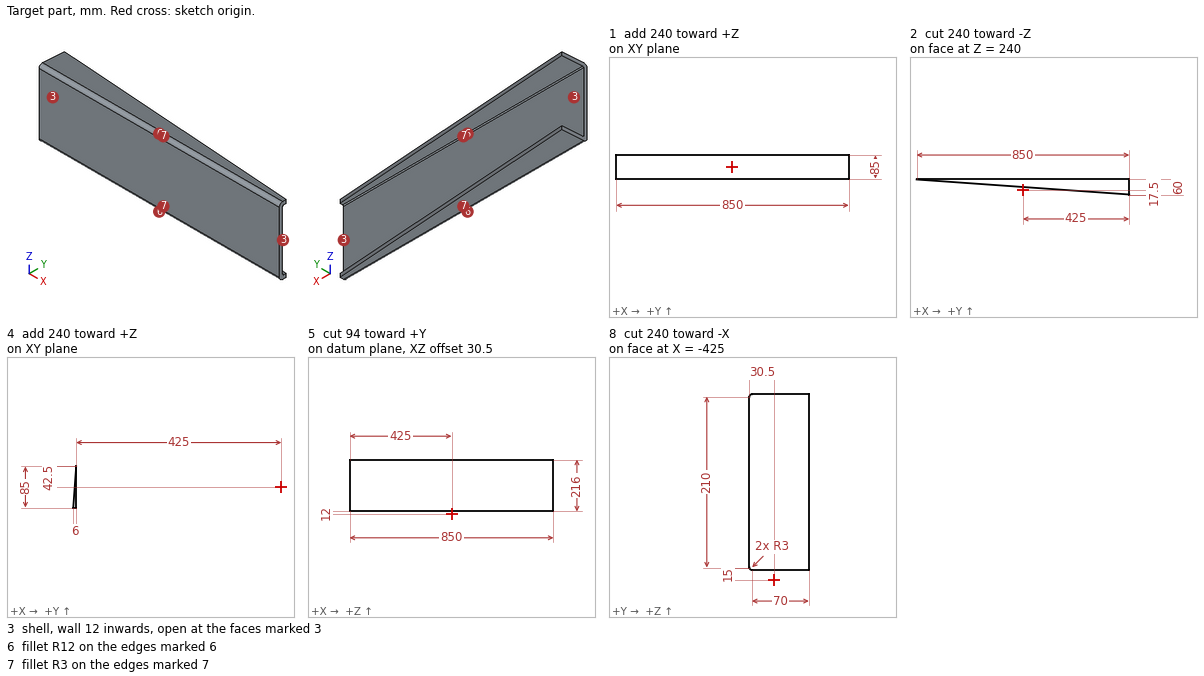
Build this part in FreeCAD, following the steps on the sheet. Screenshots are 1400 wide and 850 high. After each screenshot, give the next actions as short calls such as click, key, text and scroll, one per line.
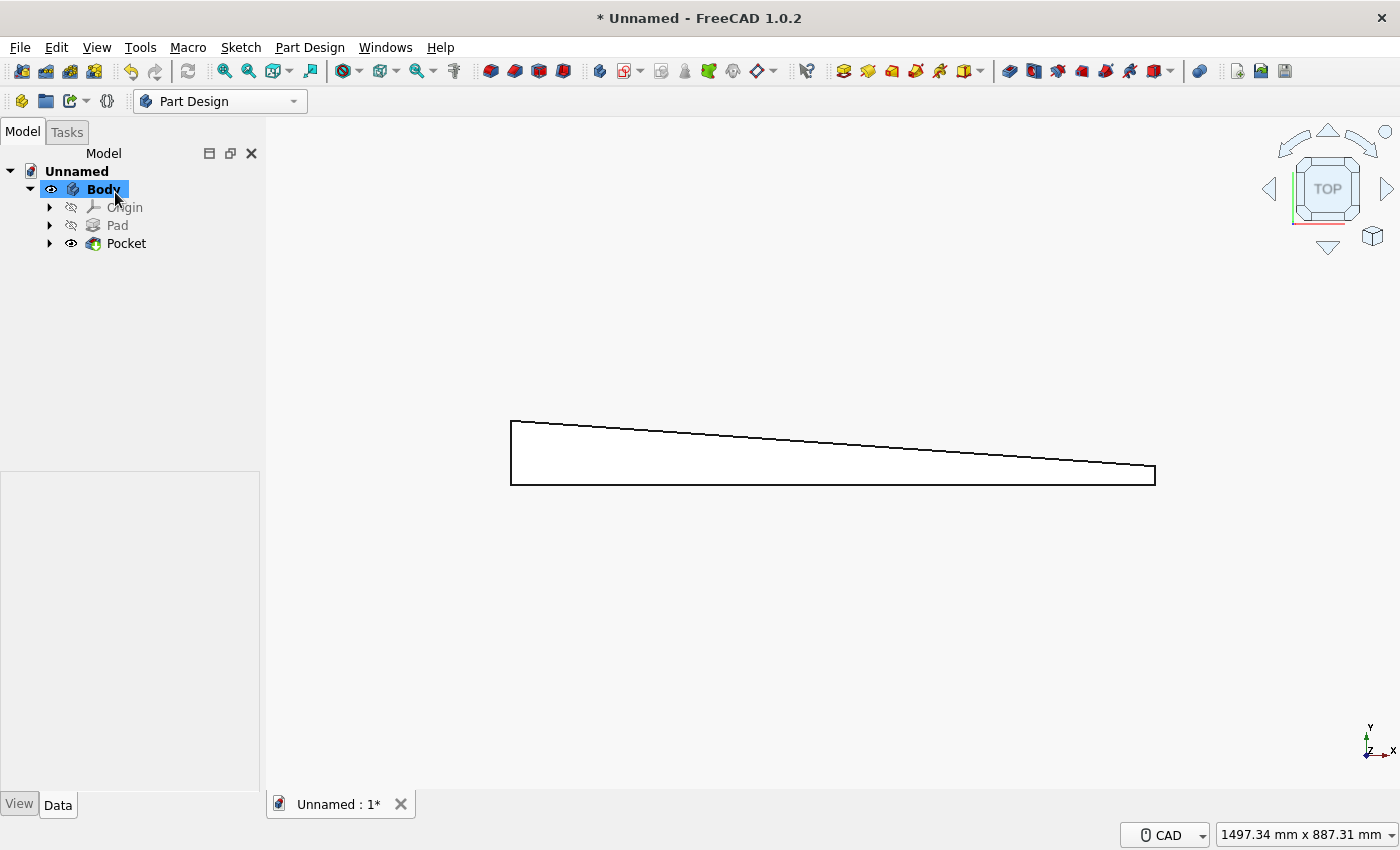
key(1)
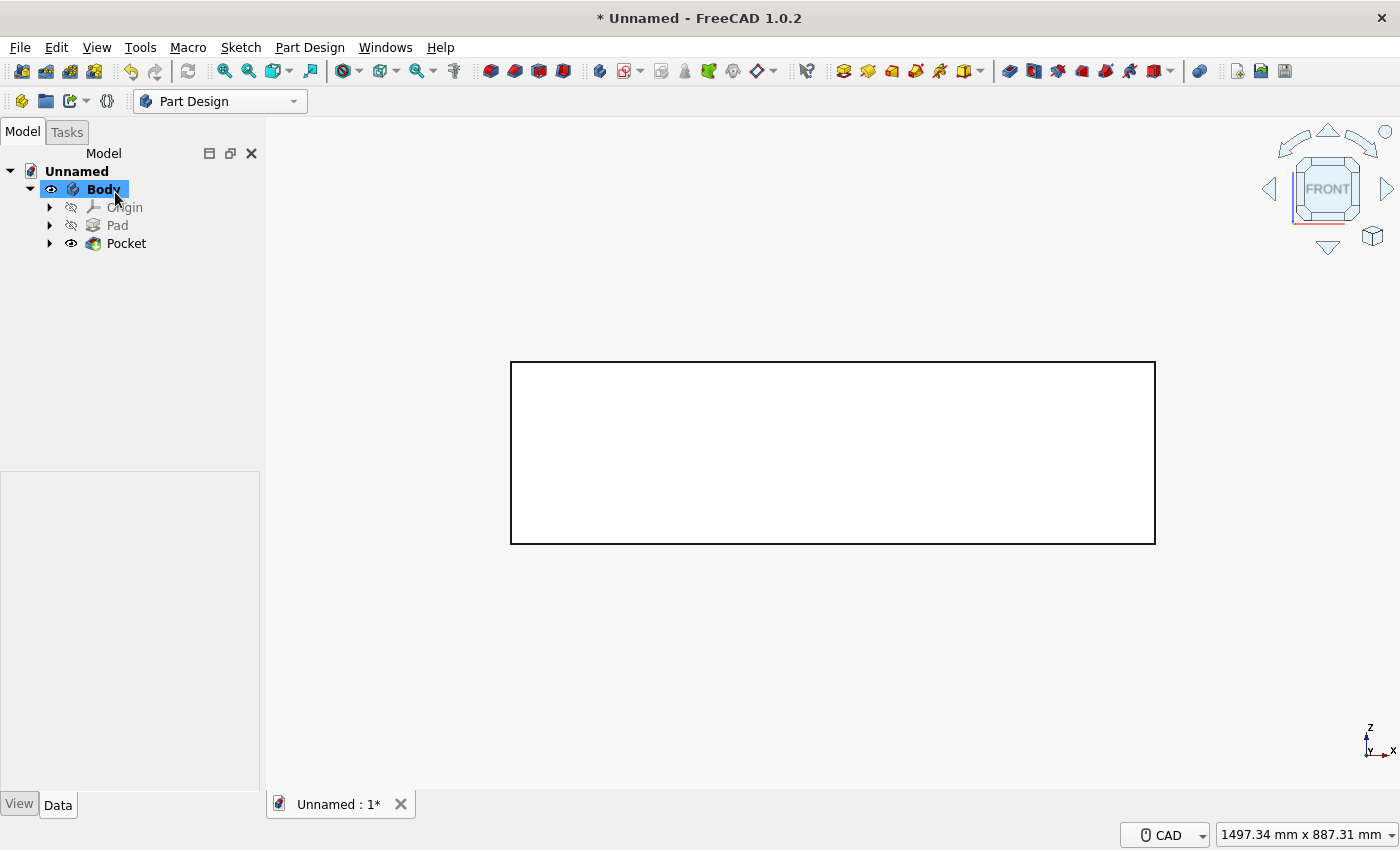
key(3)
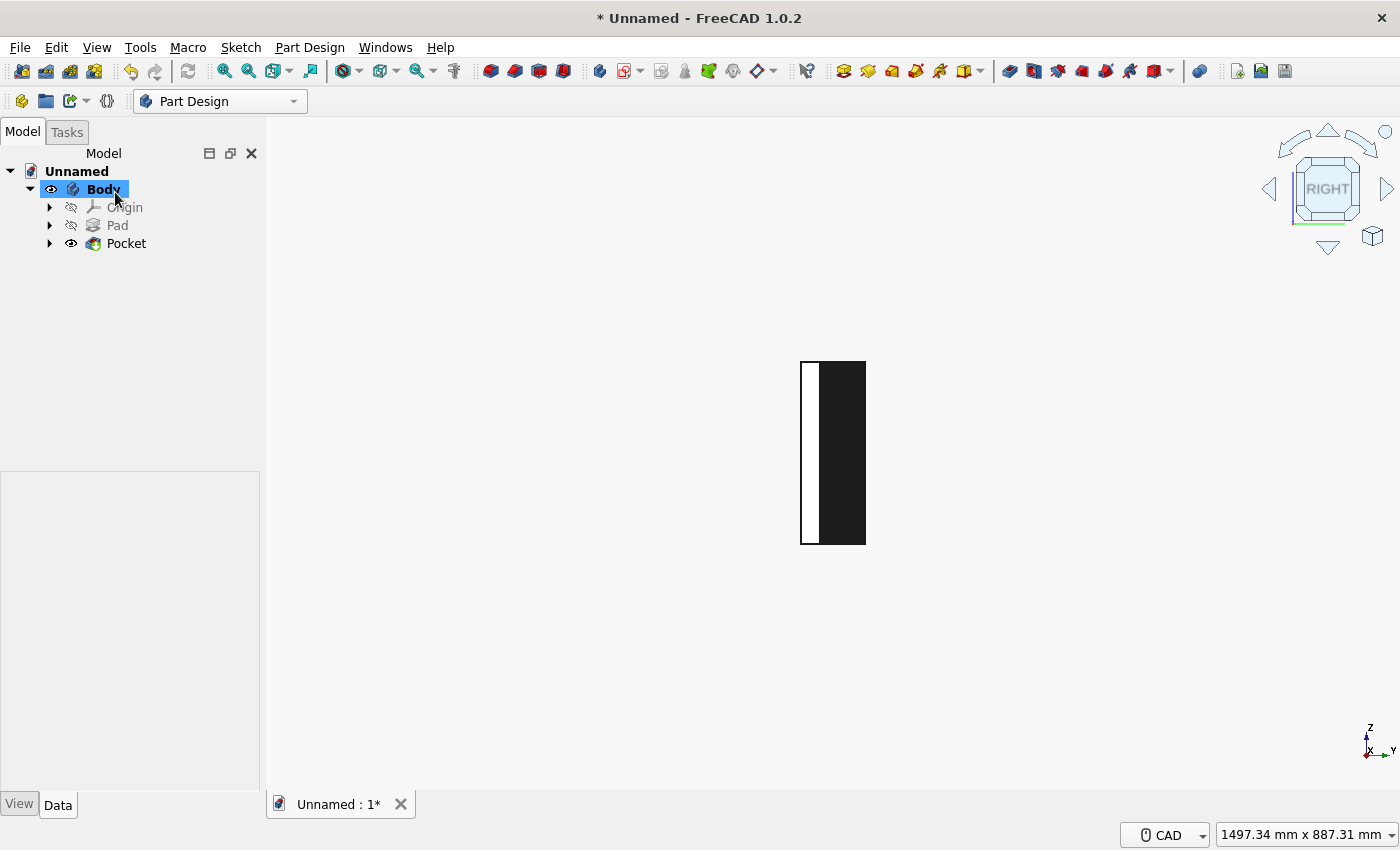
key(v)
key(f)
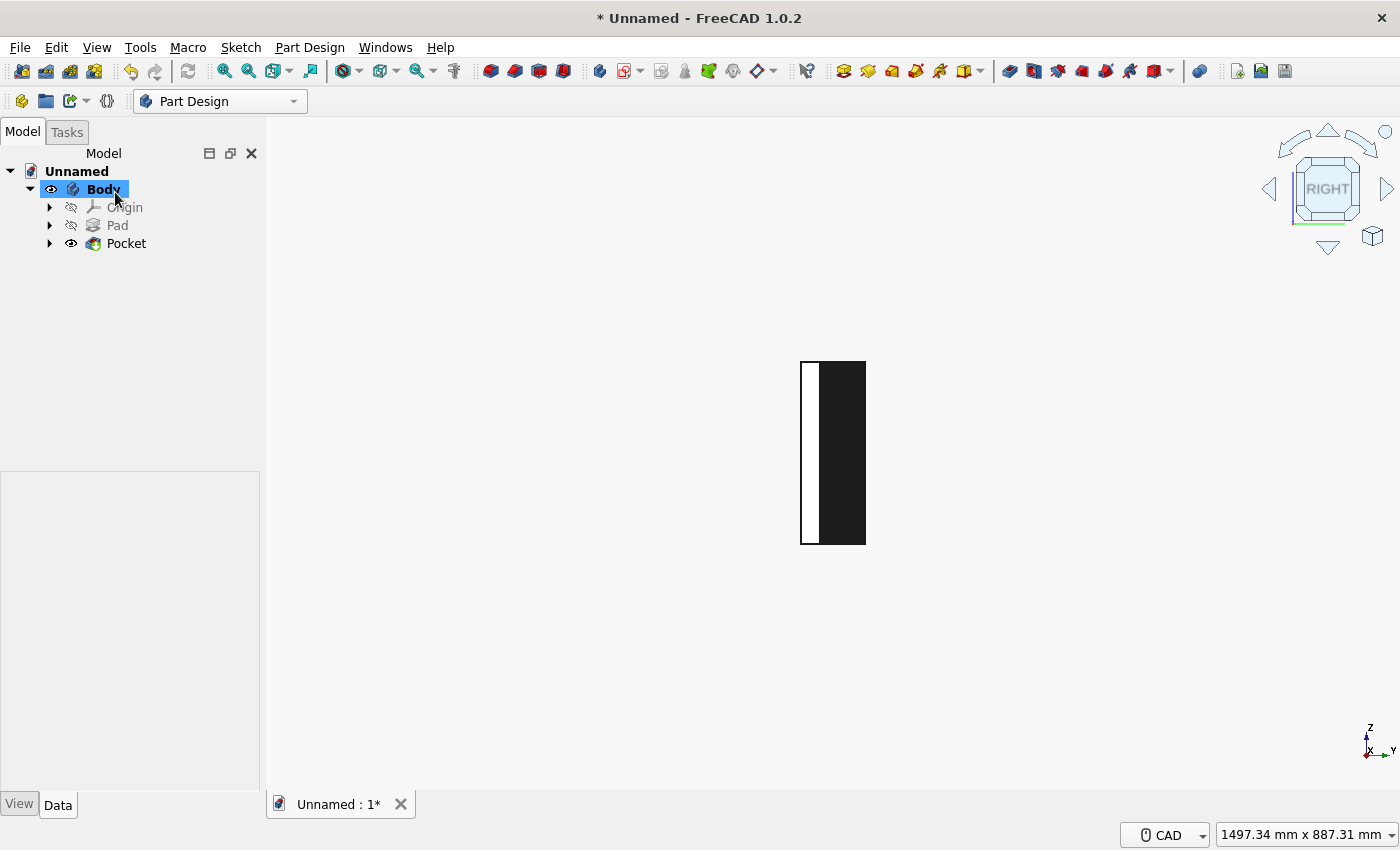
click(810, 374)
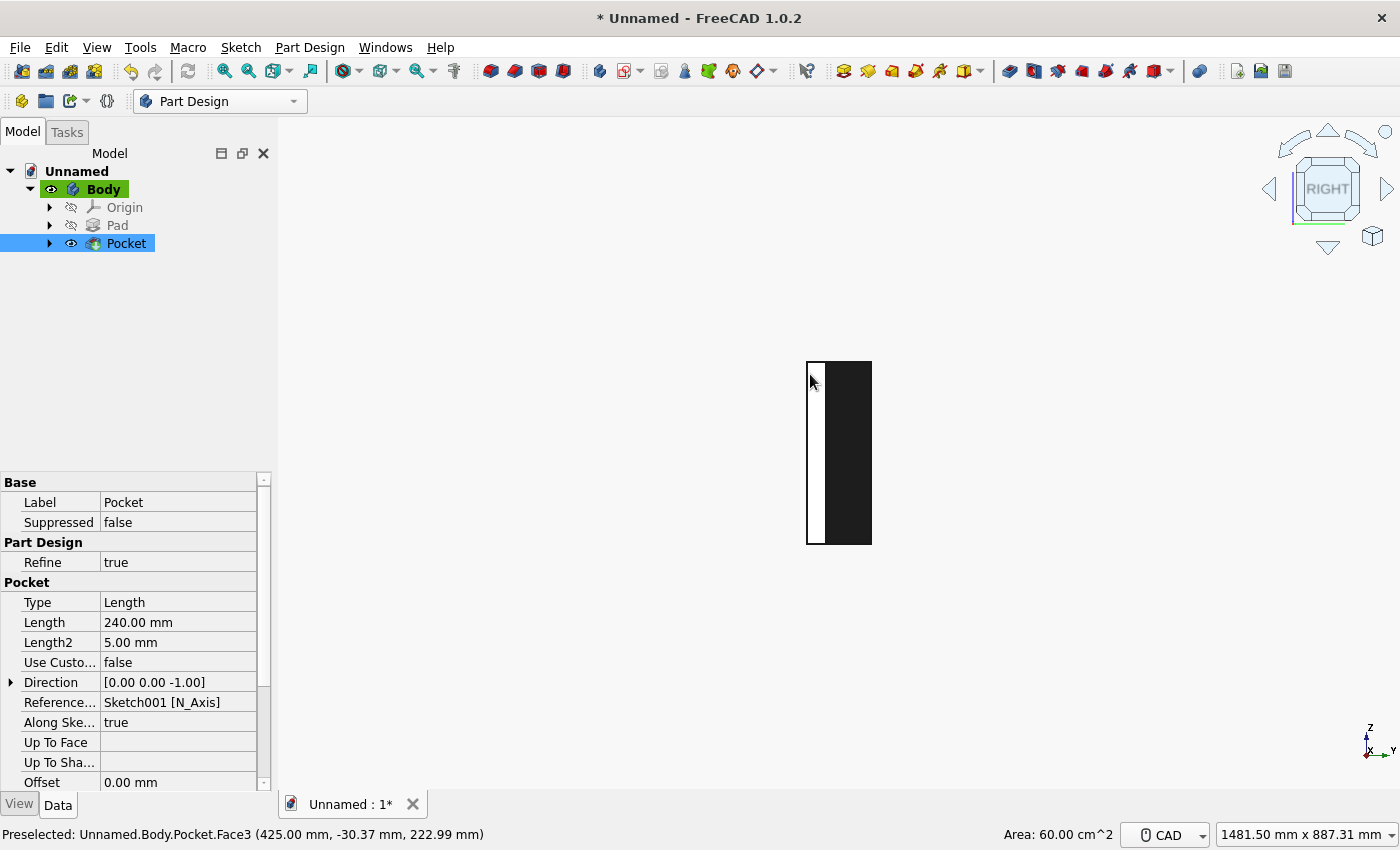
key(5)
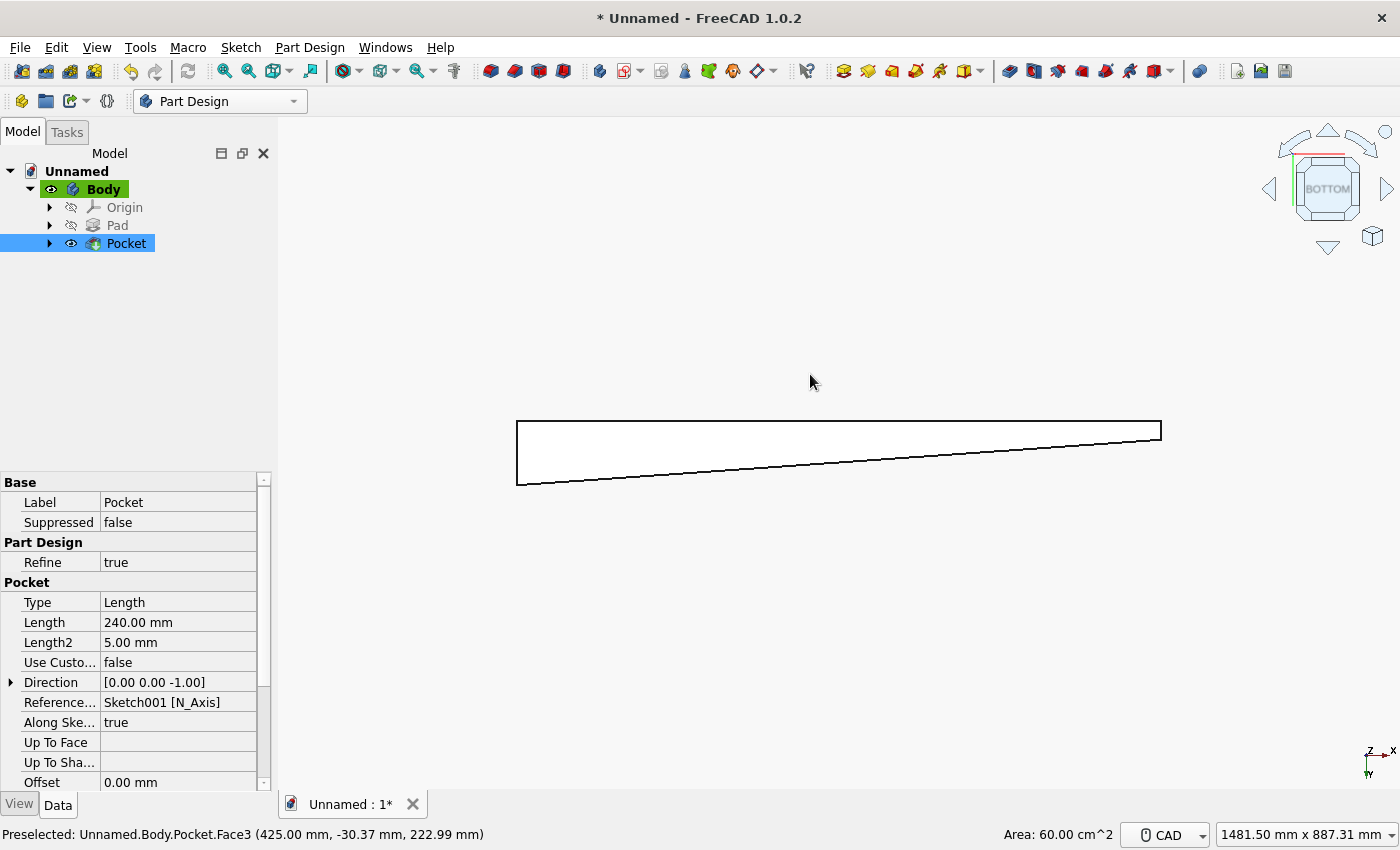
key(4)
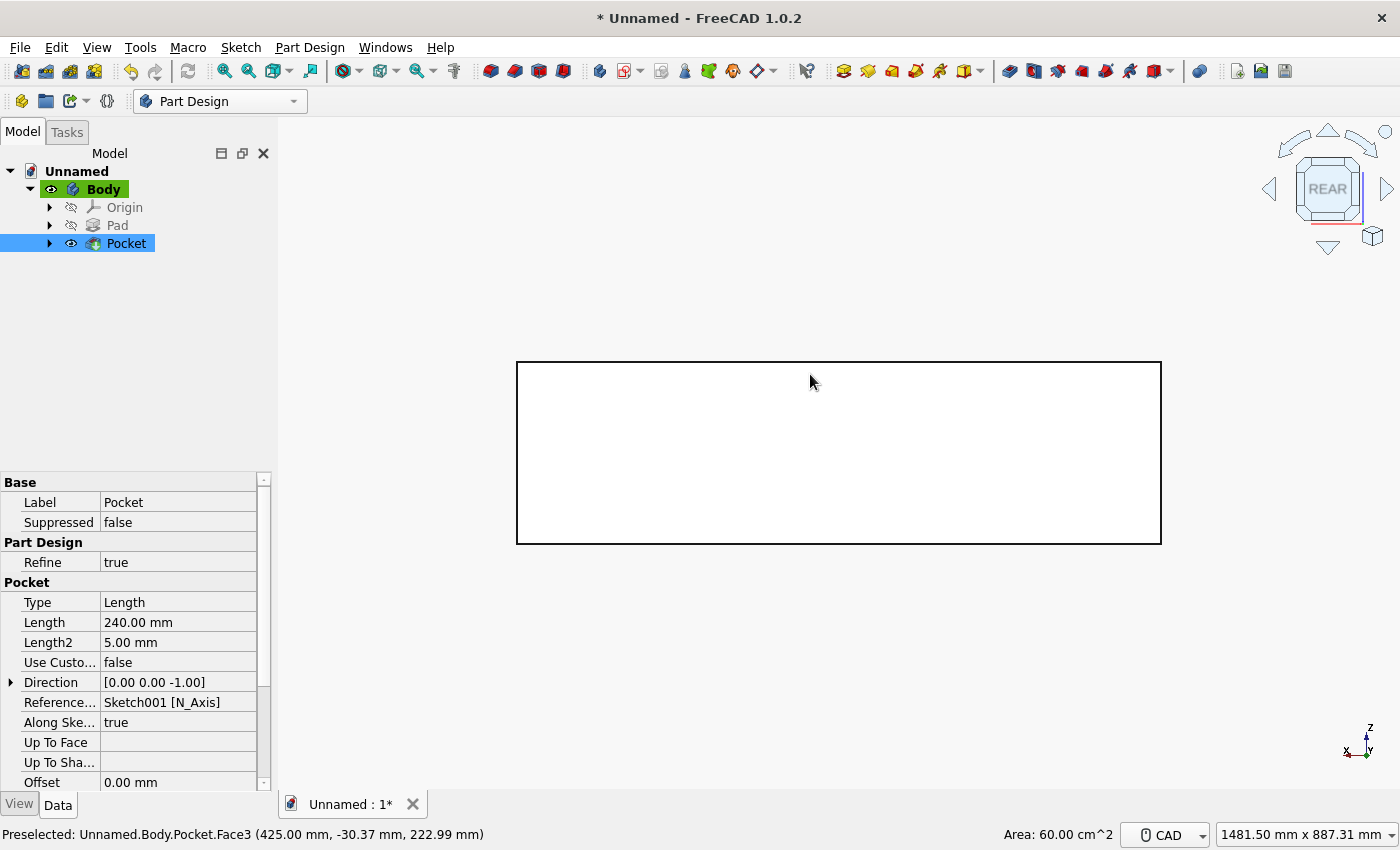
key(6)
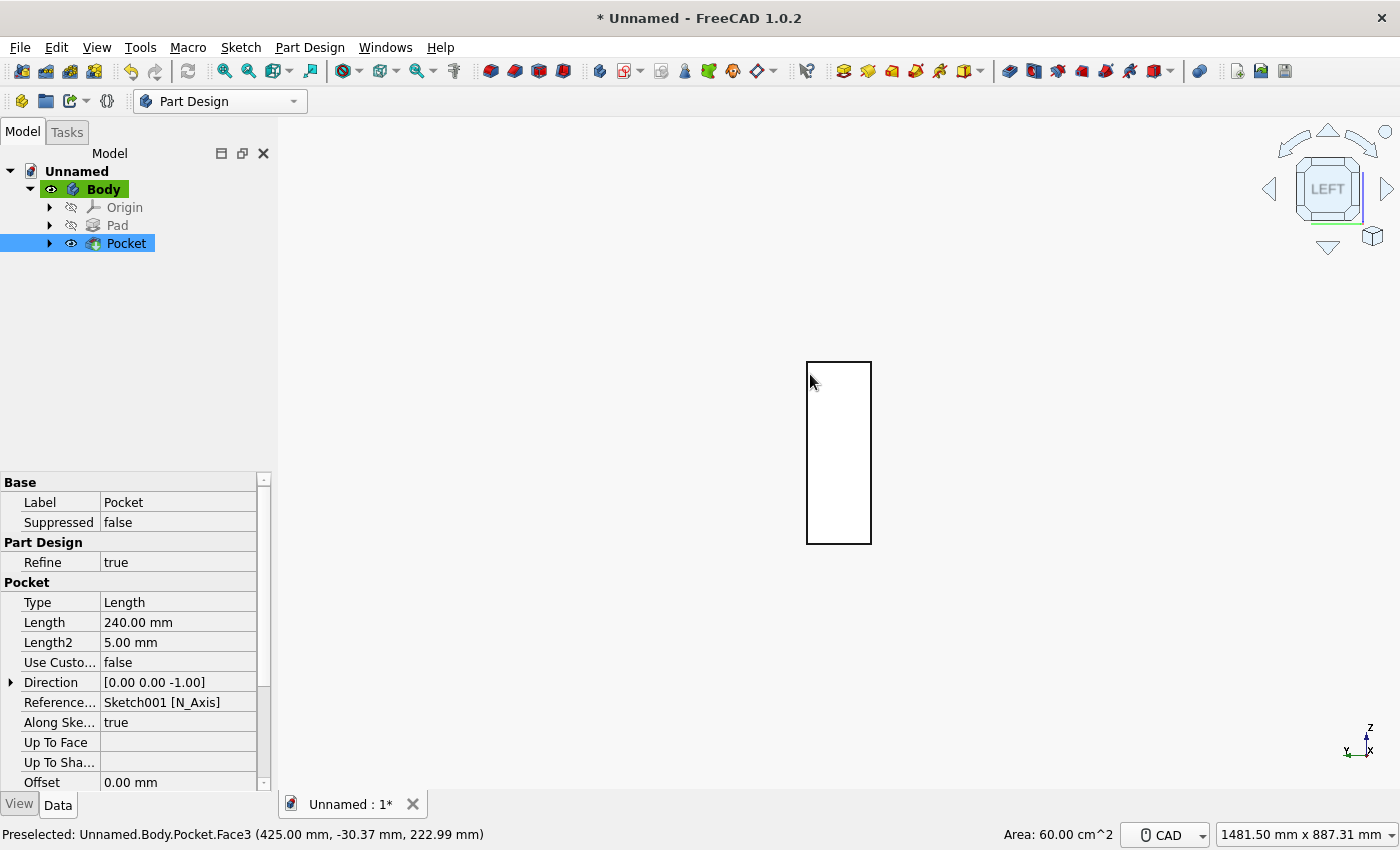
key(v)
key(f)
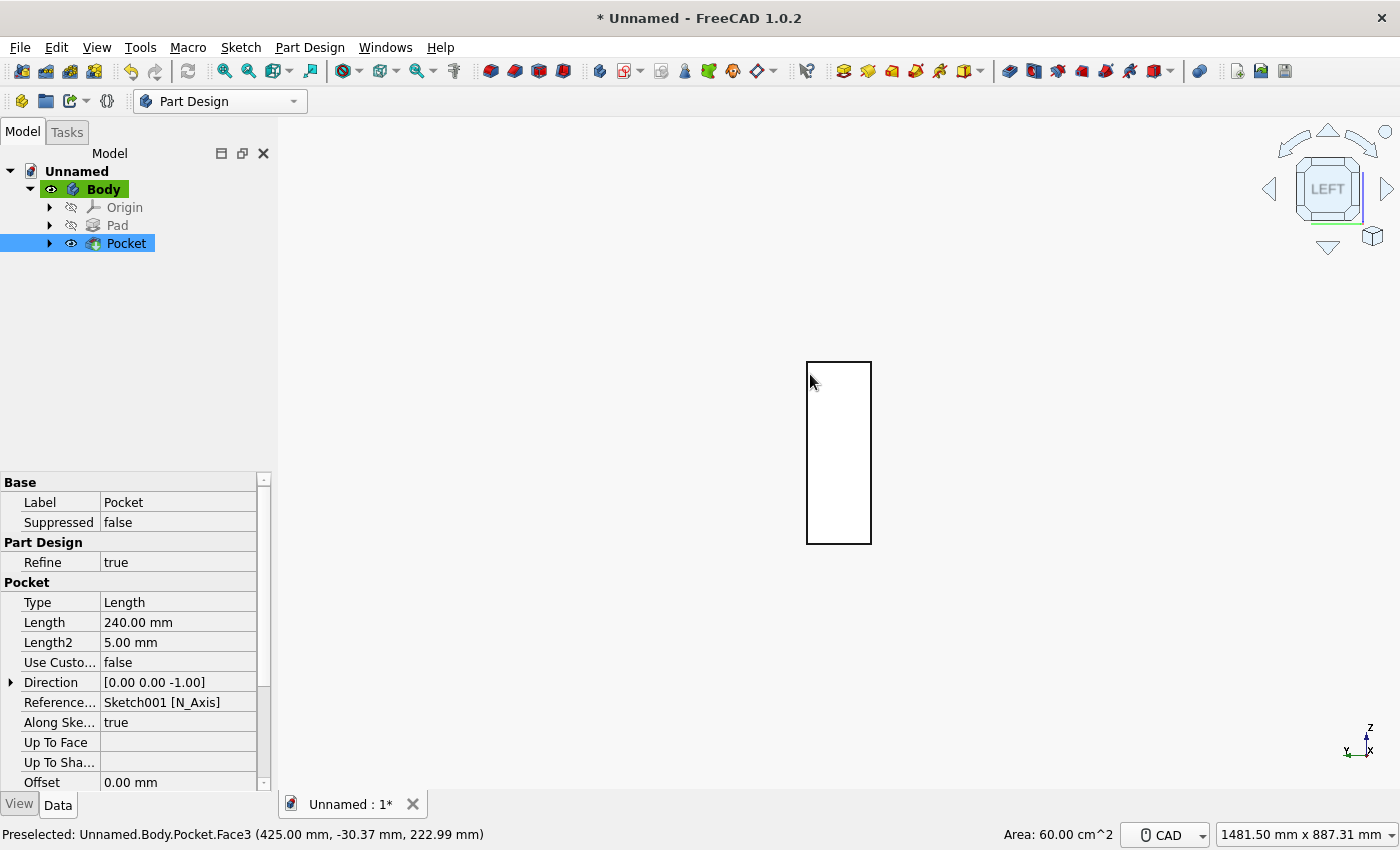
click(839, 400, ctrl)